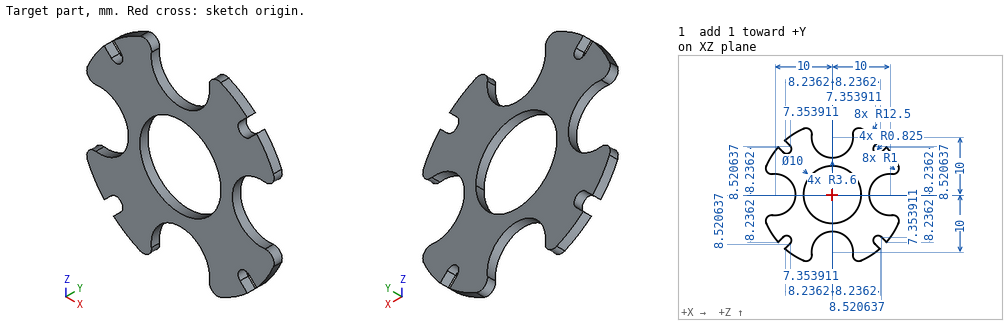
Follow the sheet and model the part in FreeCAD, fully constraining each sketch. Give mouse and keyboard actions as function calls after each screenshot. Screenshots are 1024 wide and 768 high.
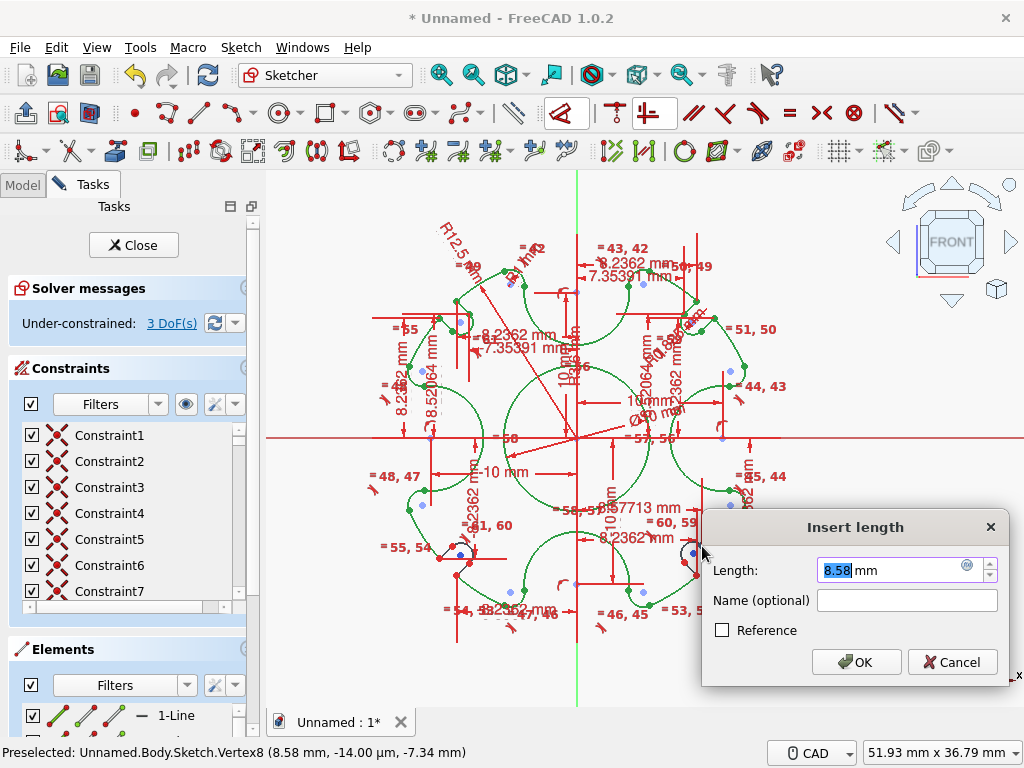
text(8.520637)
key(Return)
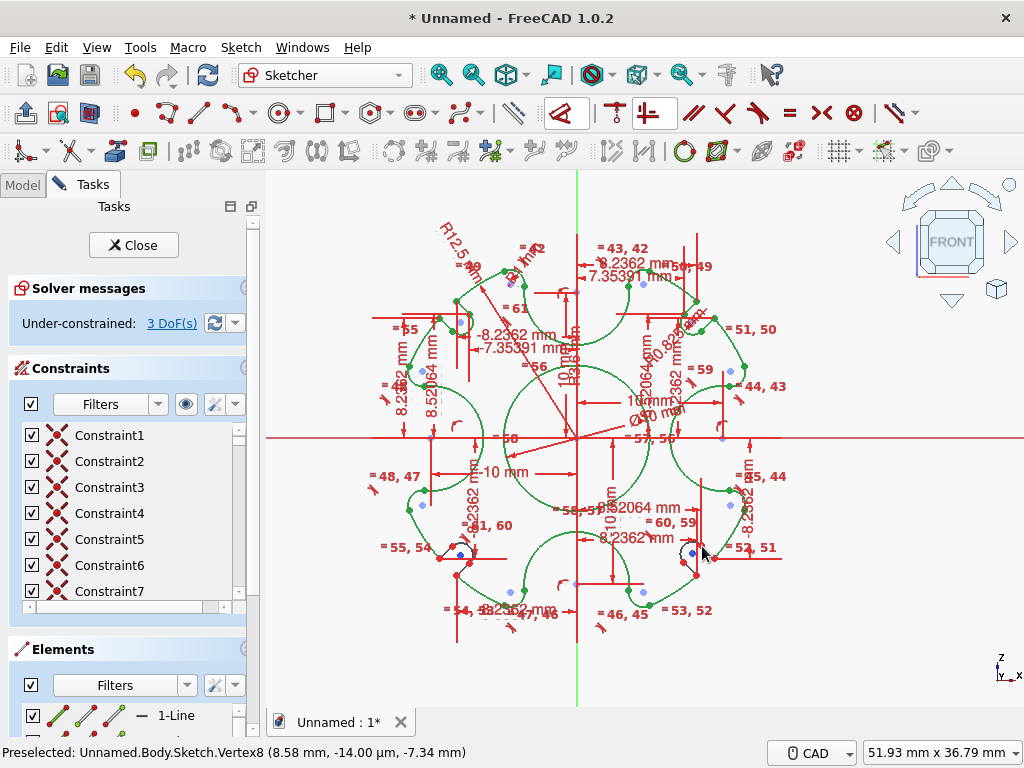
click(701, 545)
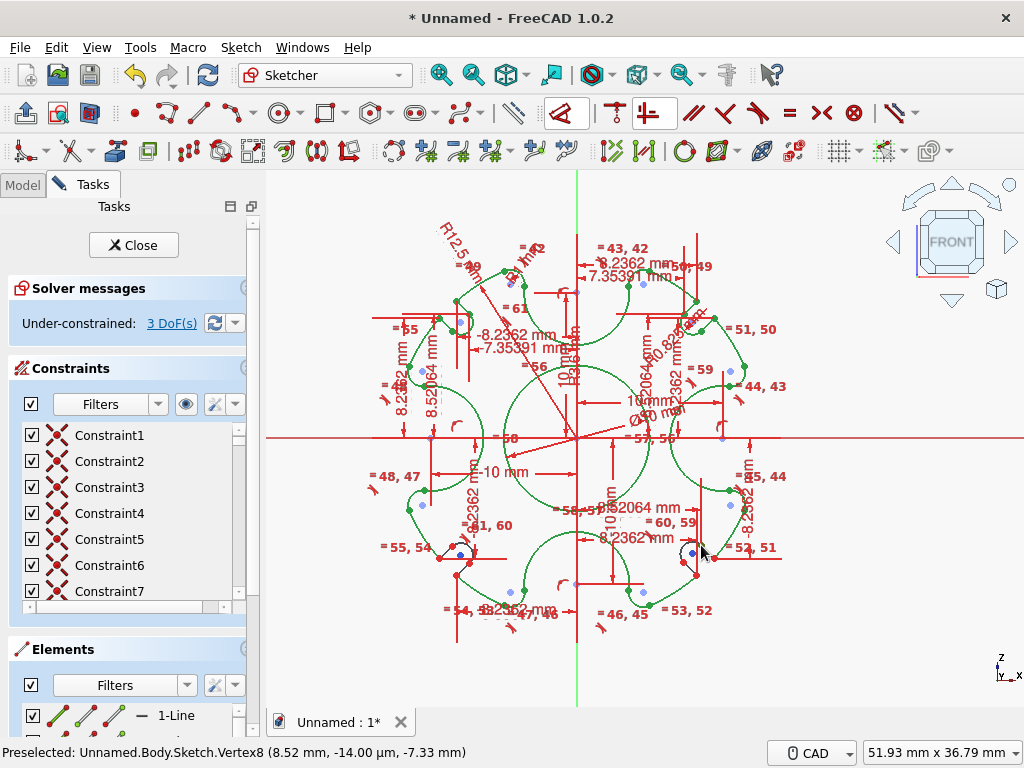
key(i)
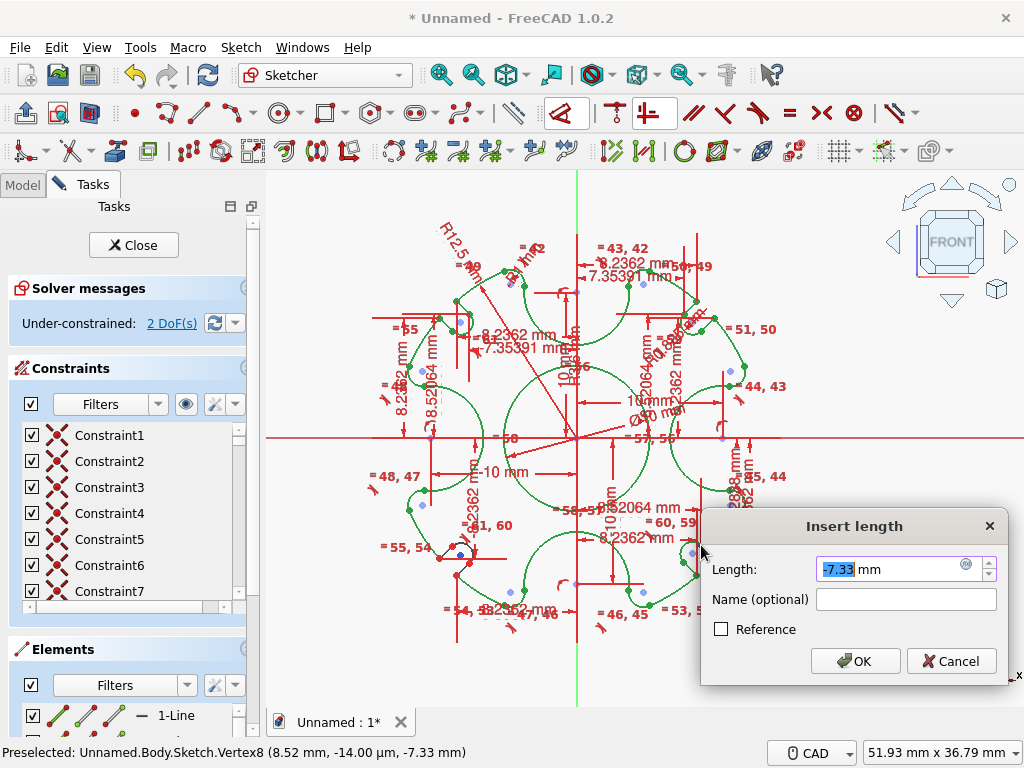
text(-7.353911)
key(Return)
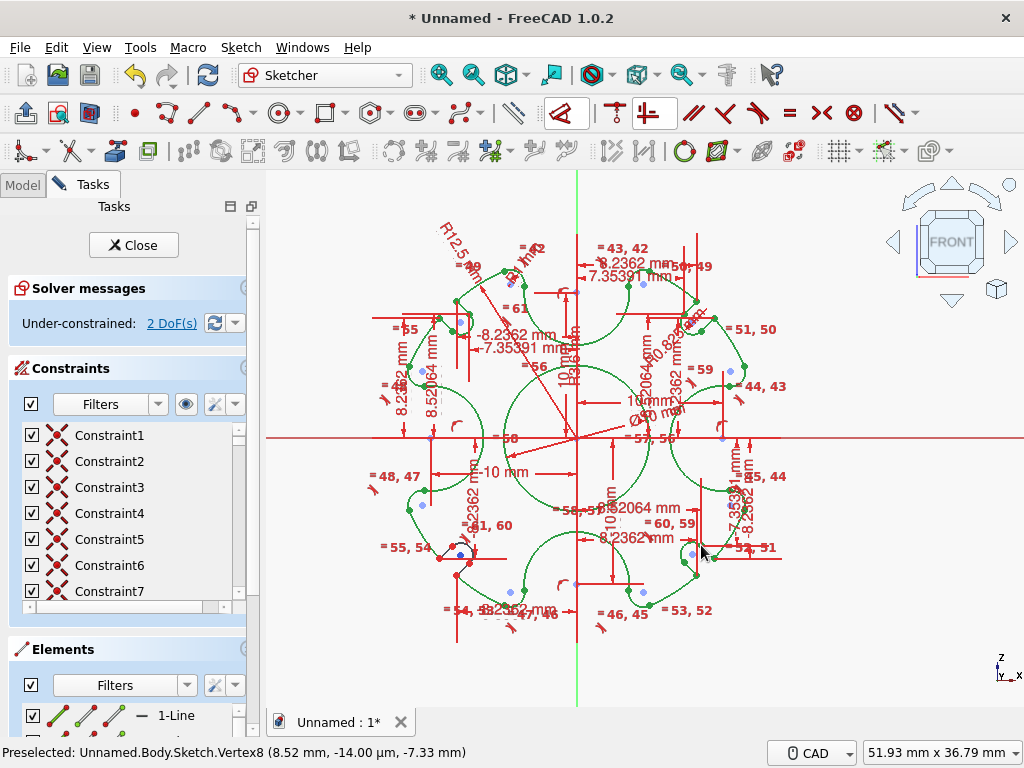
click(469, 564)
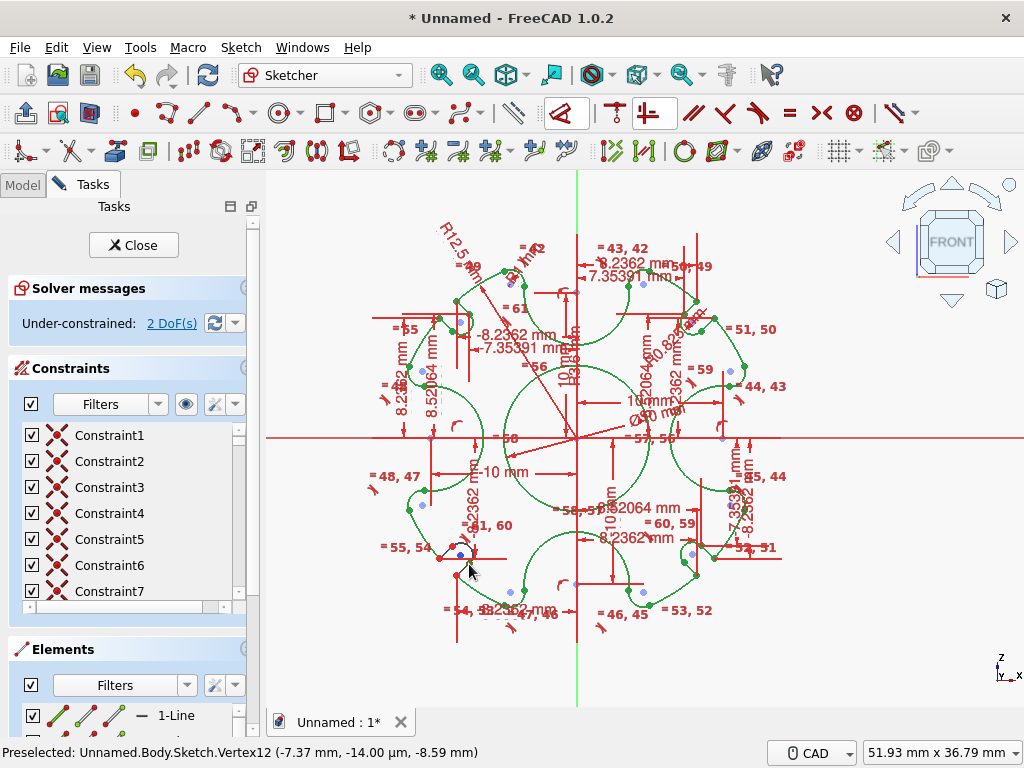
key(l)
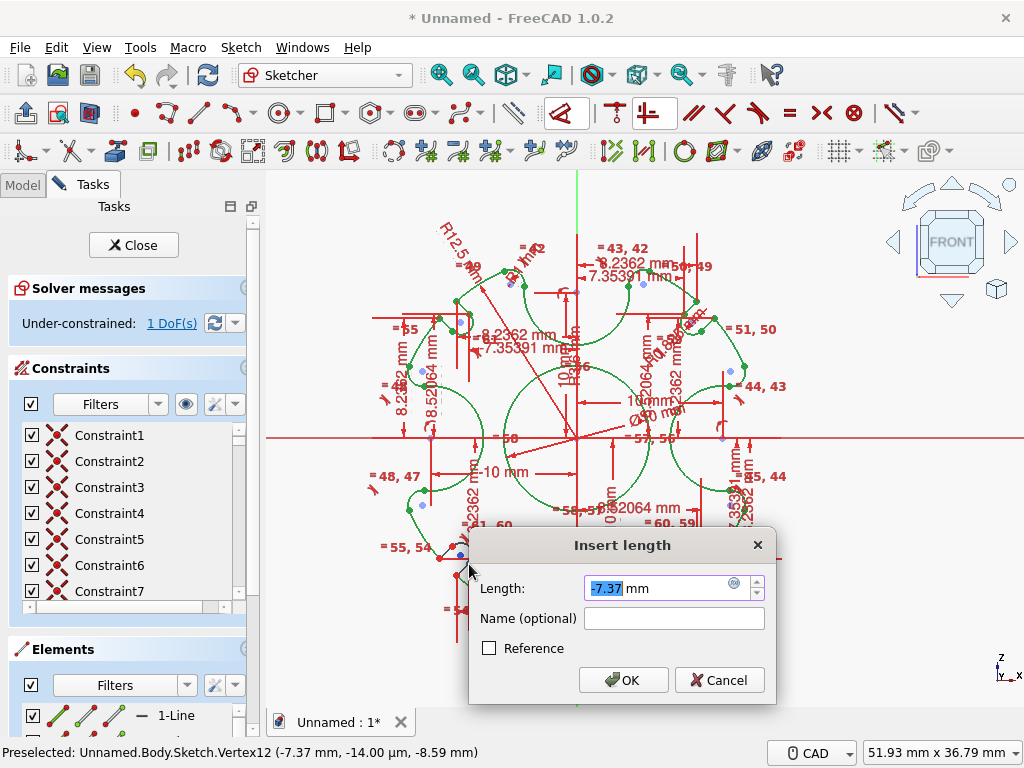
text(-7.353911)
key(Return)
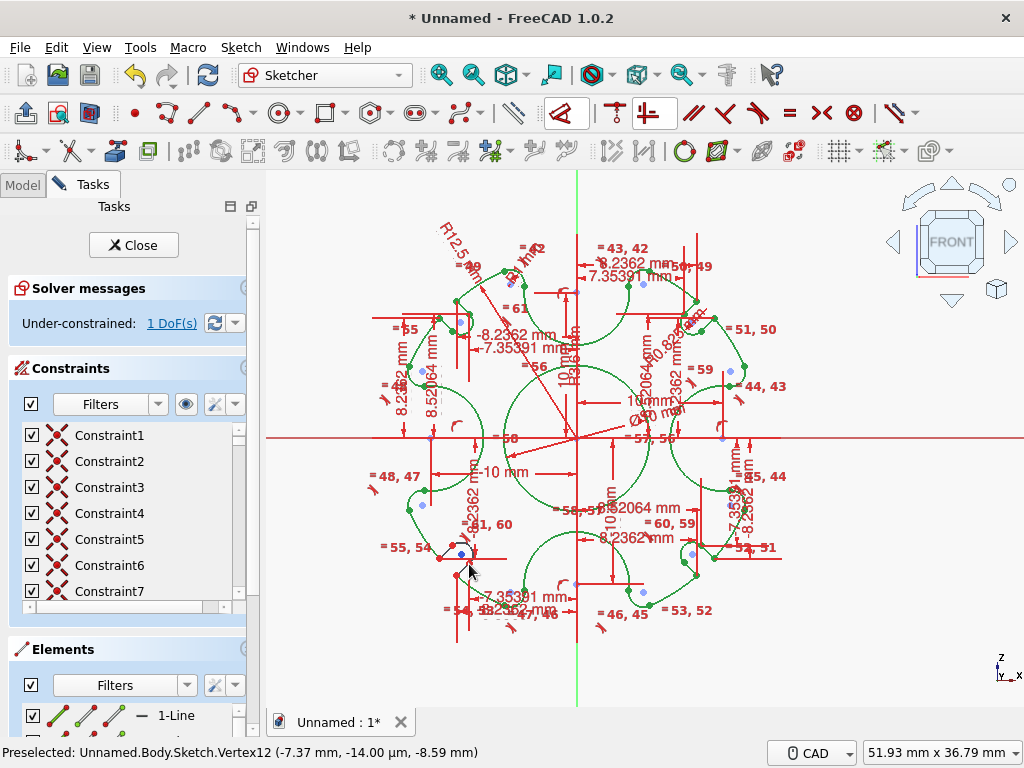
click(469, 563)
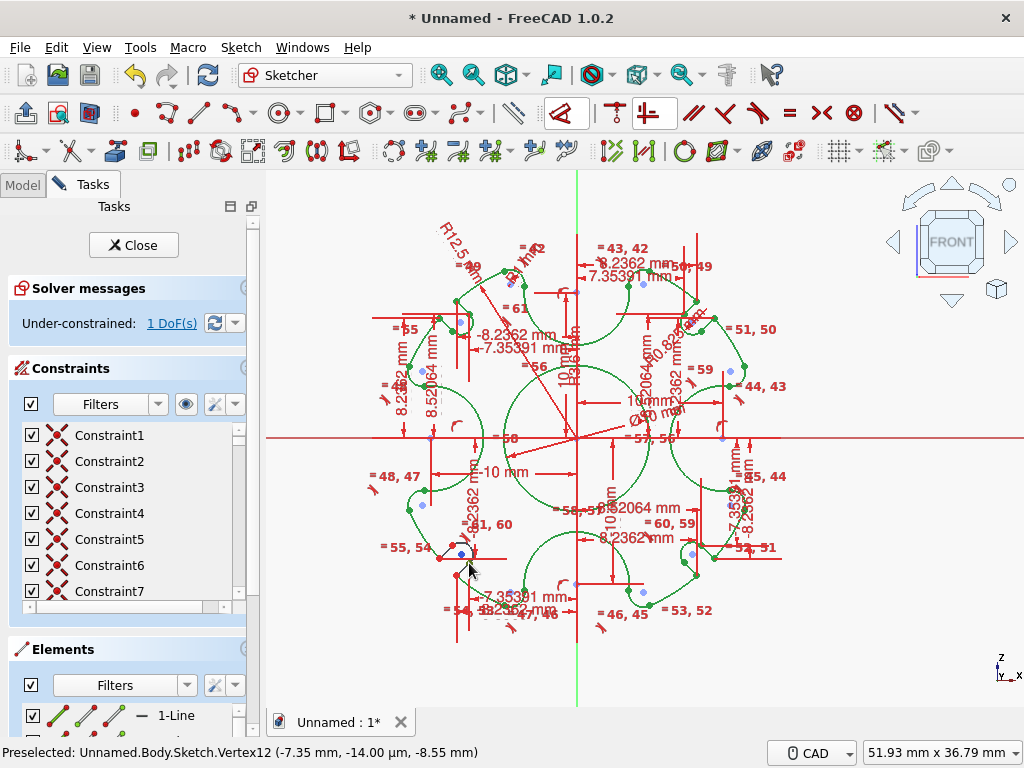
key(i)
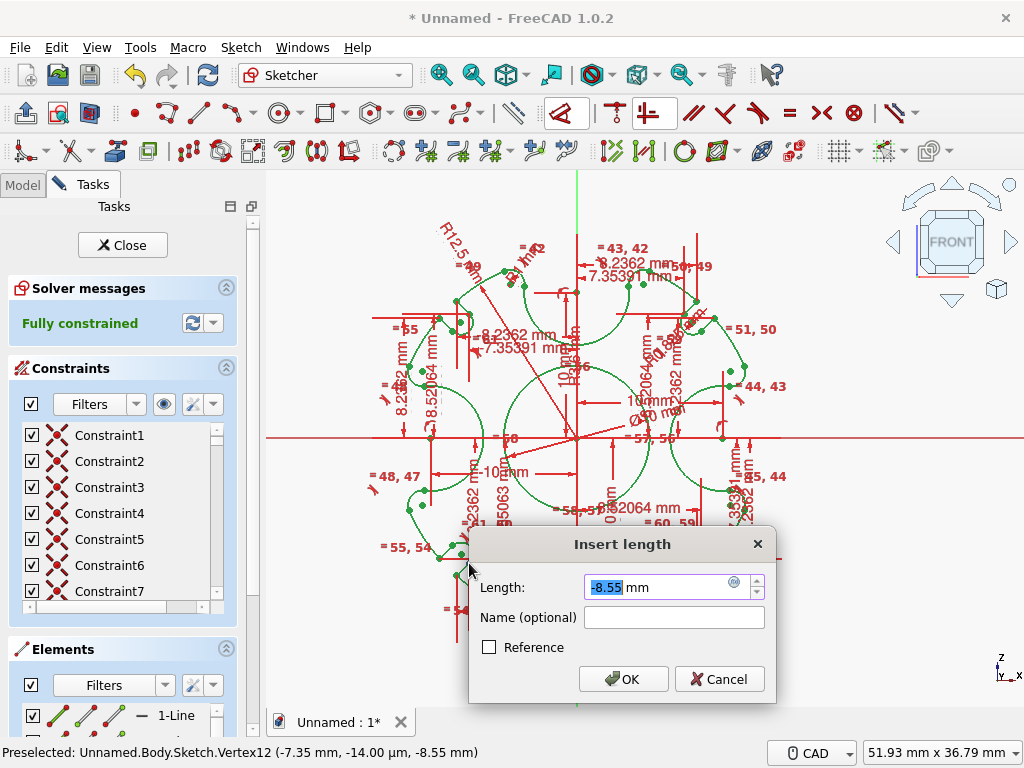
text(-8.520637)
key(Return)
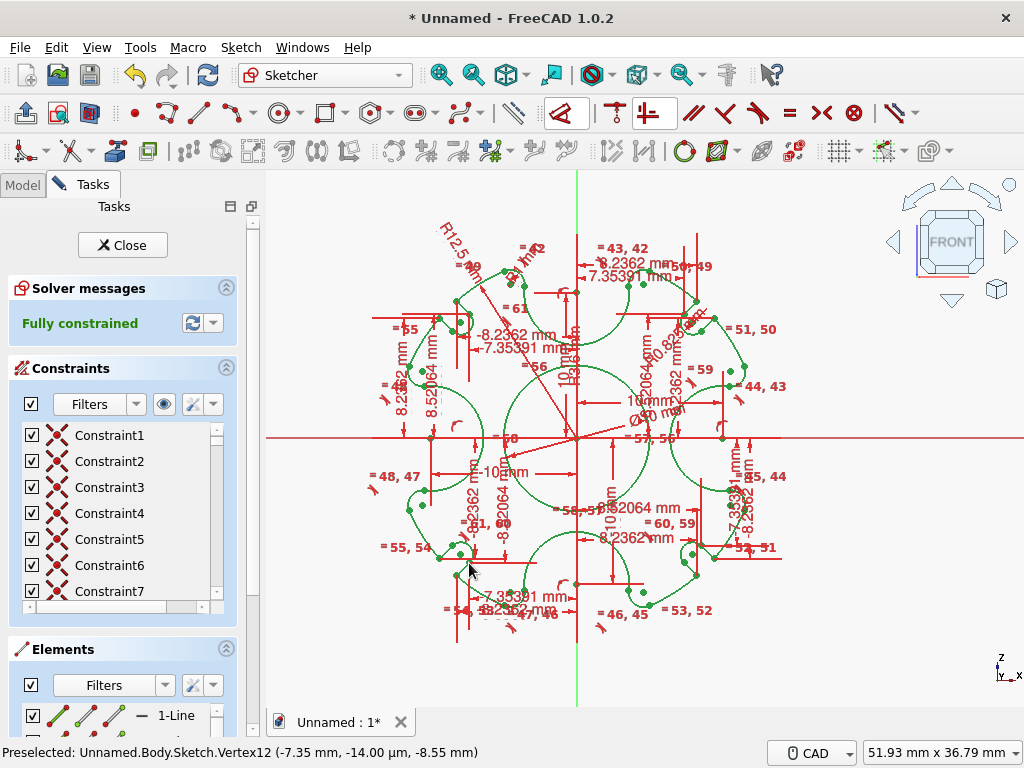
click(123, 245)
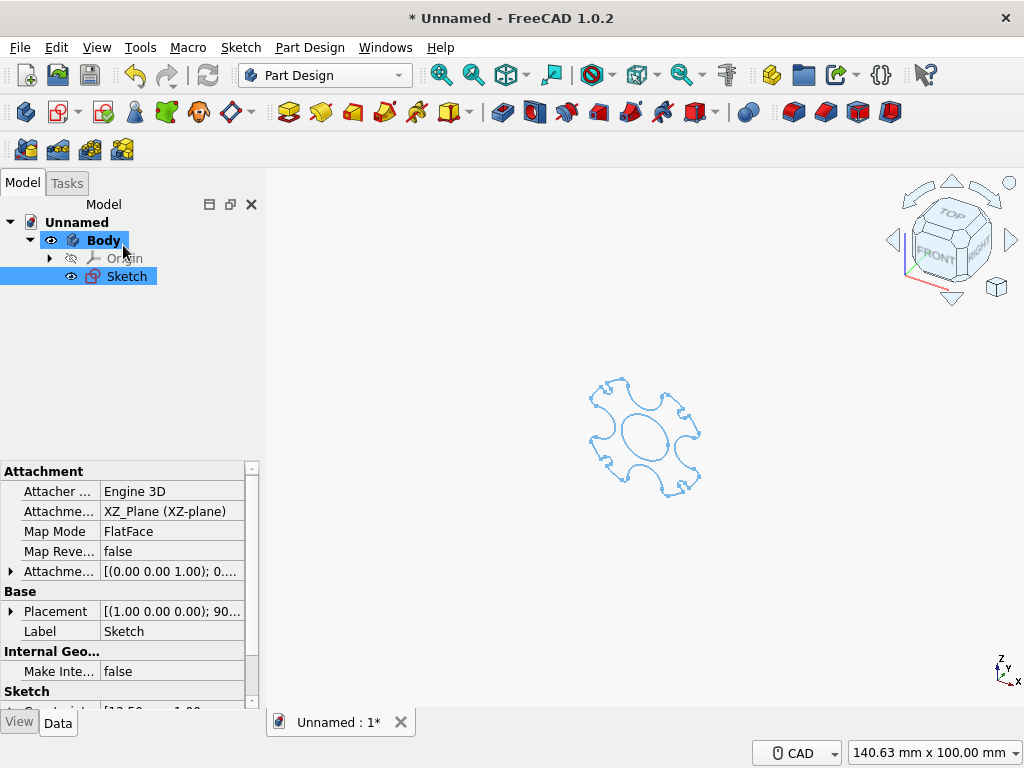
click(290, 112)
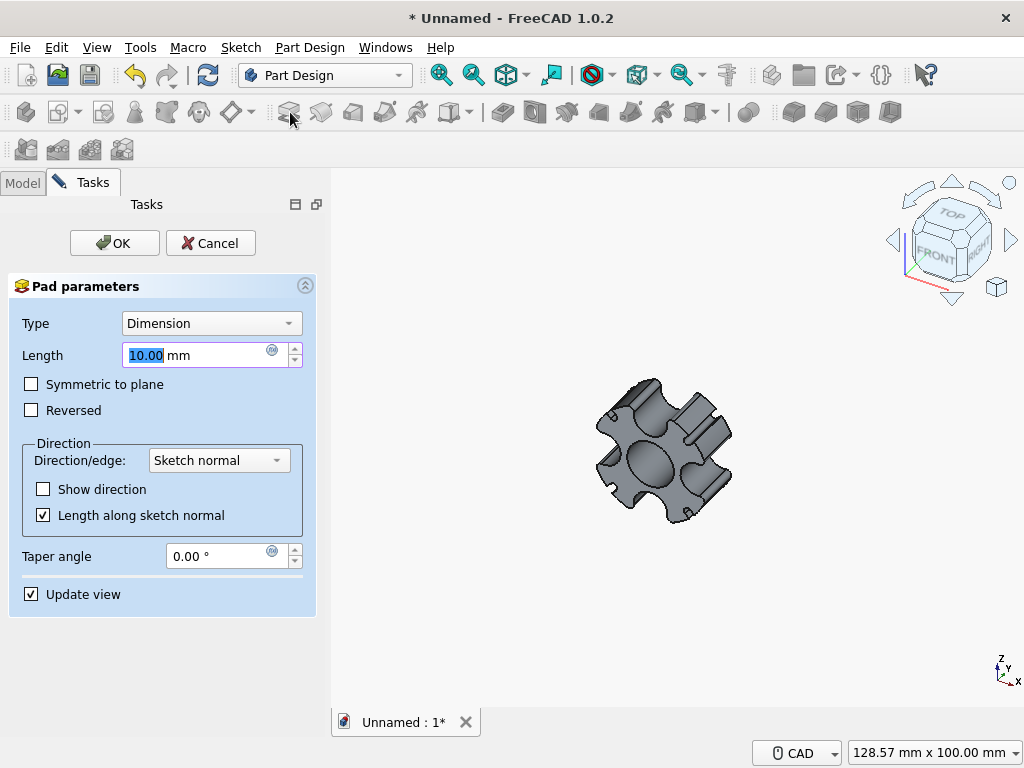
text(1)
key(Tab)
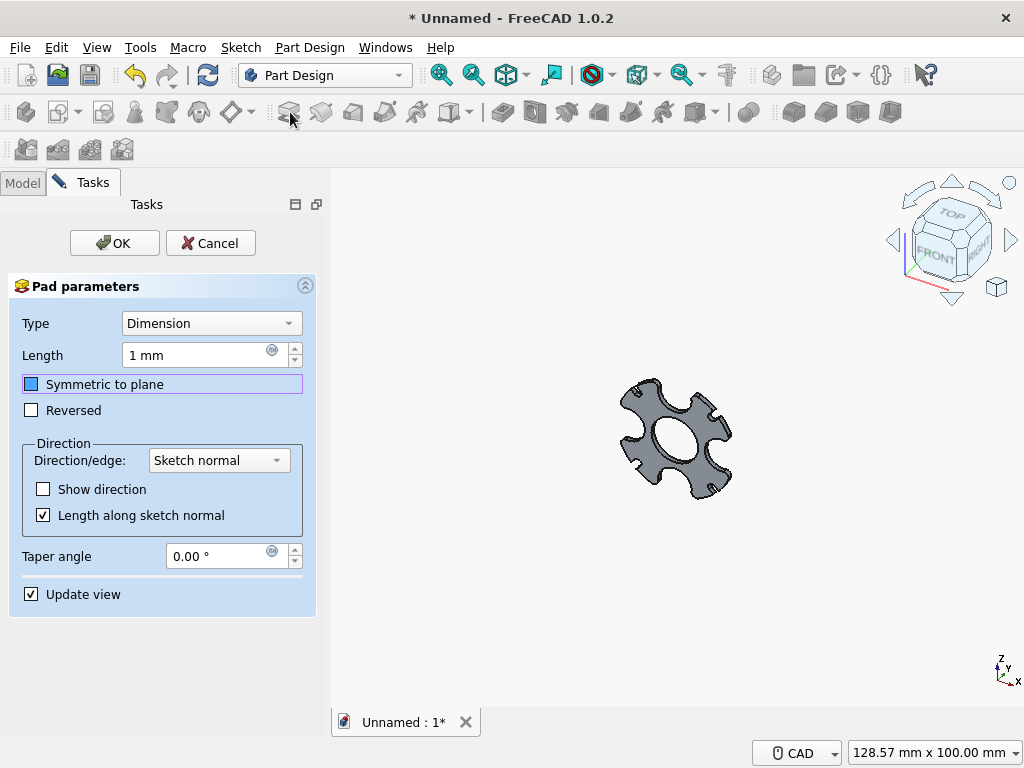
click(30, 410)